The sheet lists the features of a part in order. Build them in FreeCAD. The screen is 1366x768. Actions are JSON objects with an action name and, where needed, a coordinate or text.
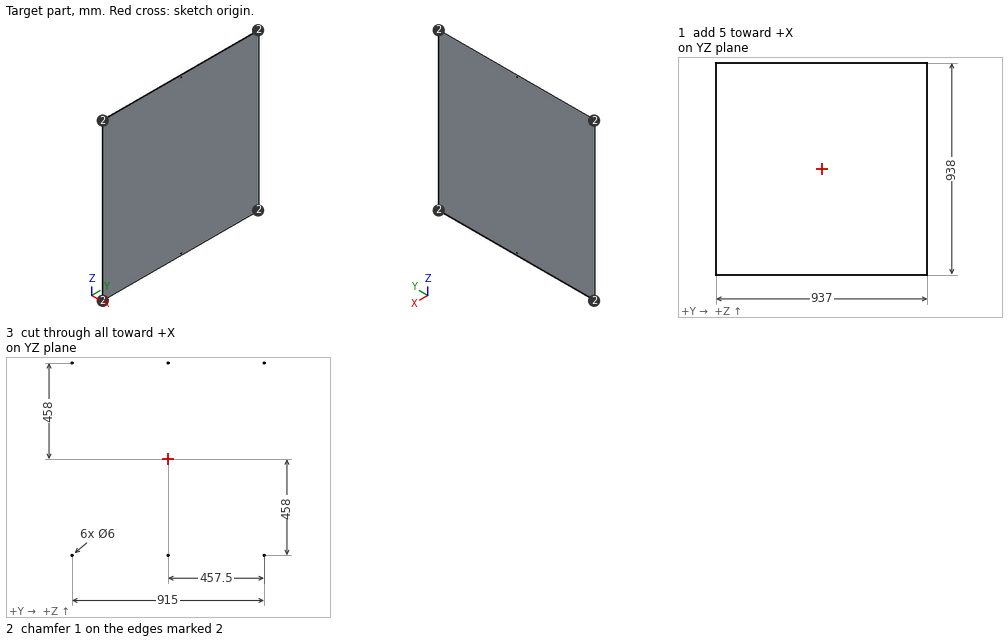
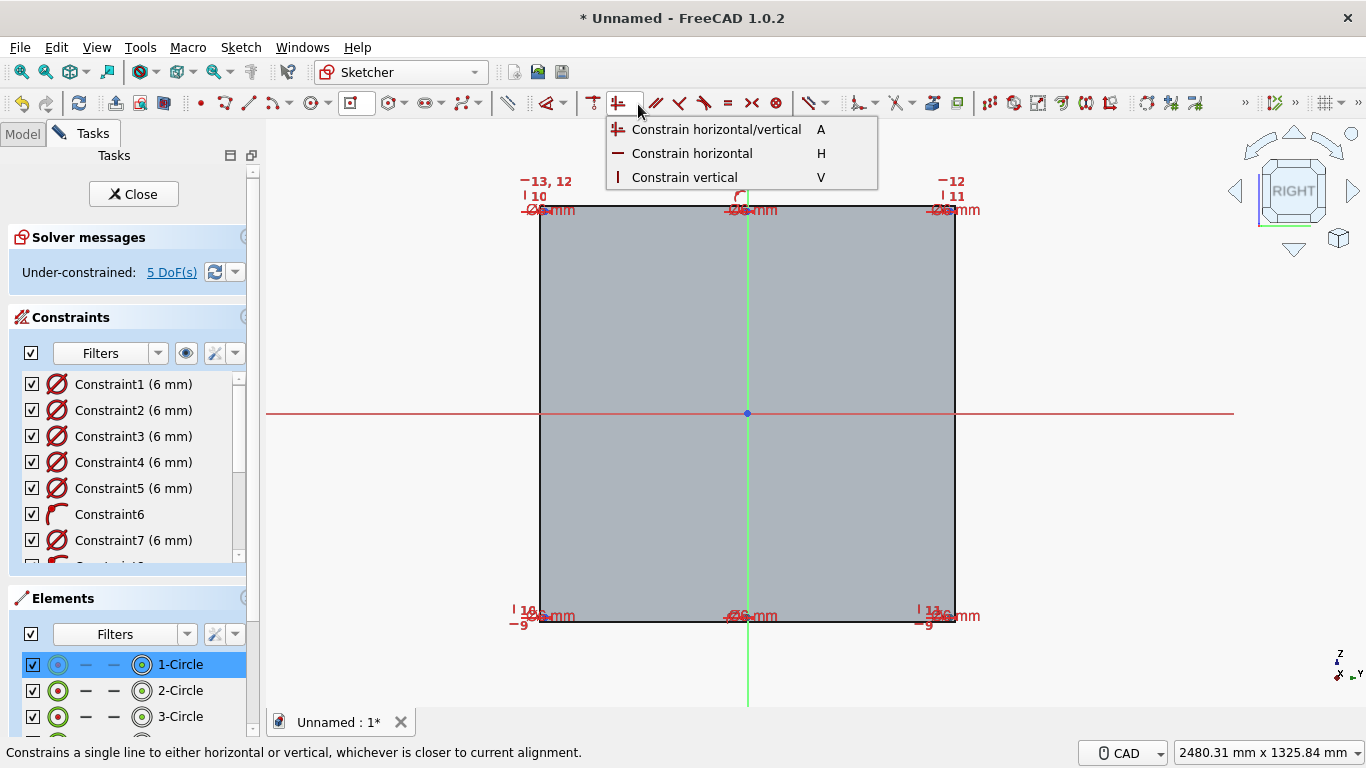
{"action": "left_click", "coordinate": [742, 153]}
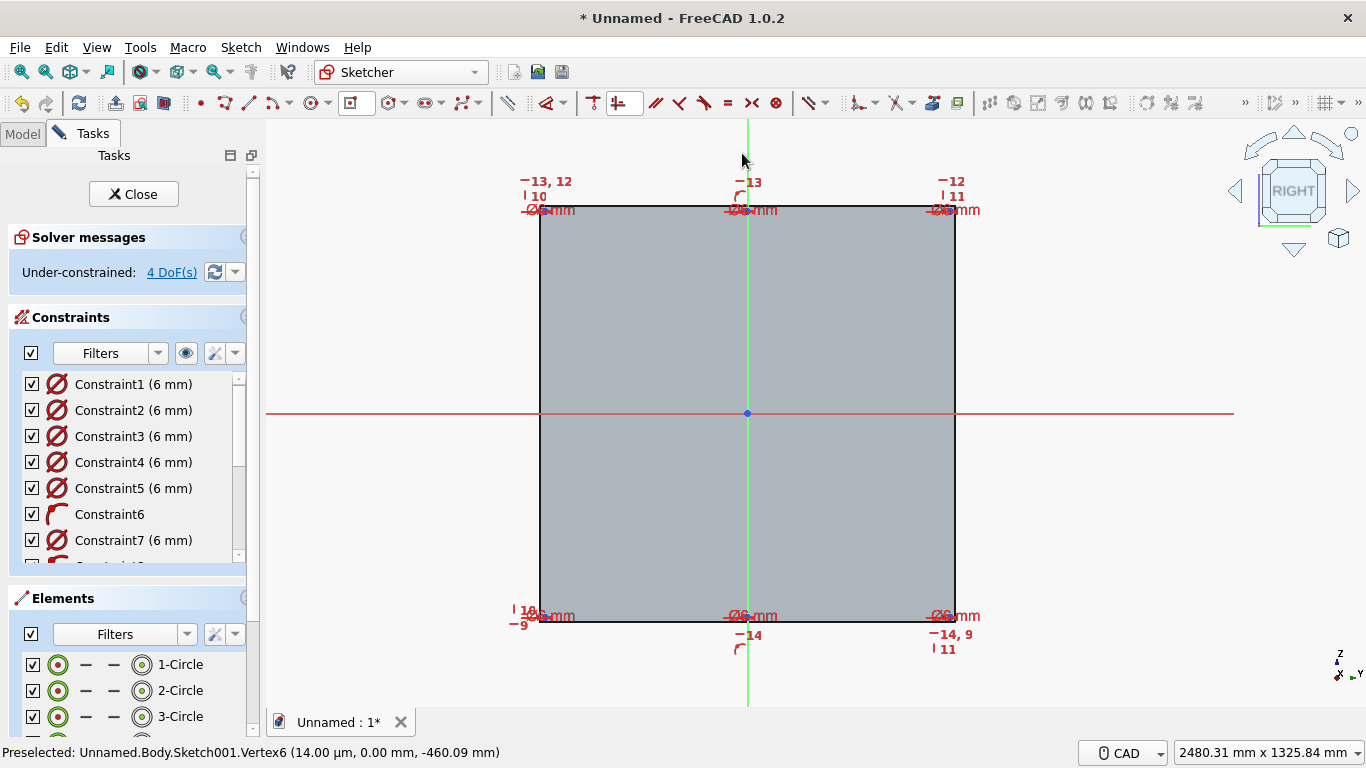
{"action": "left_click", "coordinate": [546, 104]}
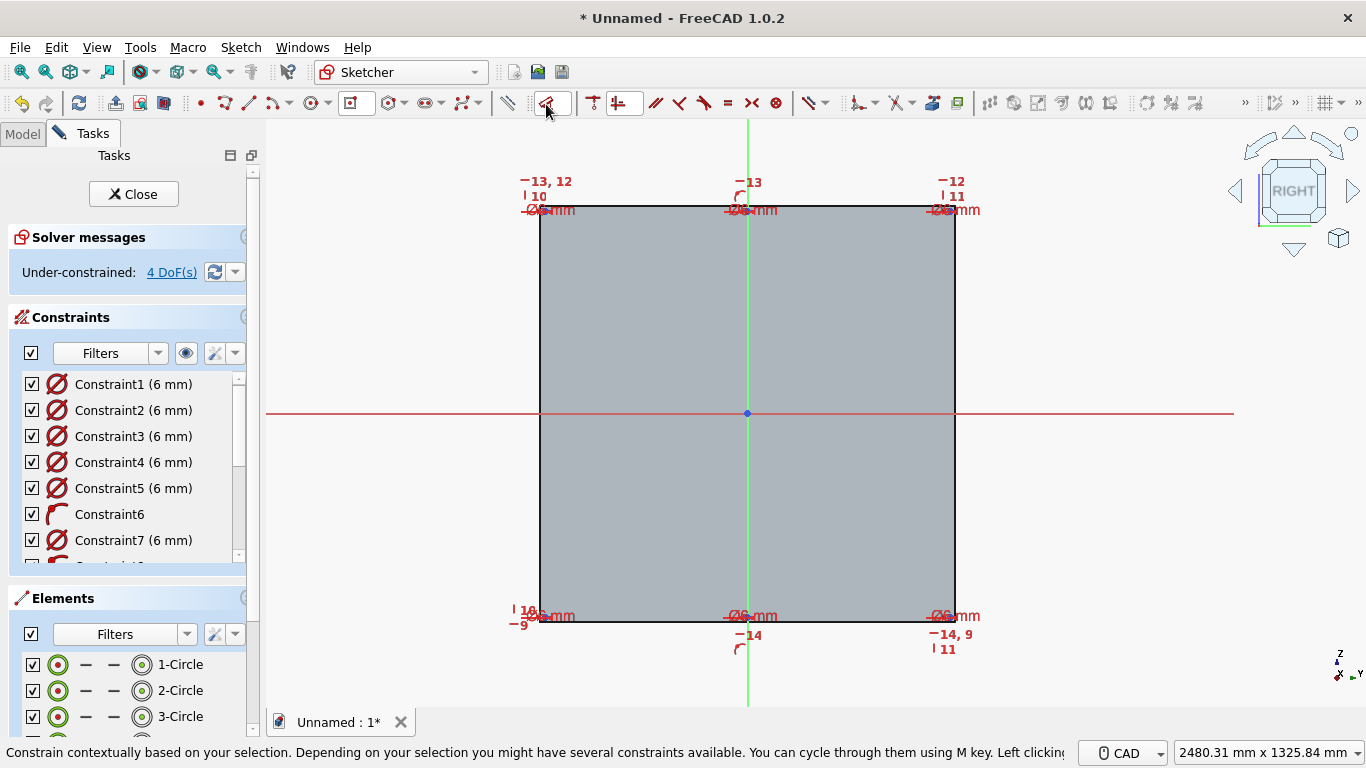
{"action": "left_click", "coordinate": [950, 618]}
{"action": "left_click", "coordinate": [984, 516]}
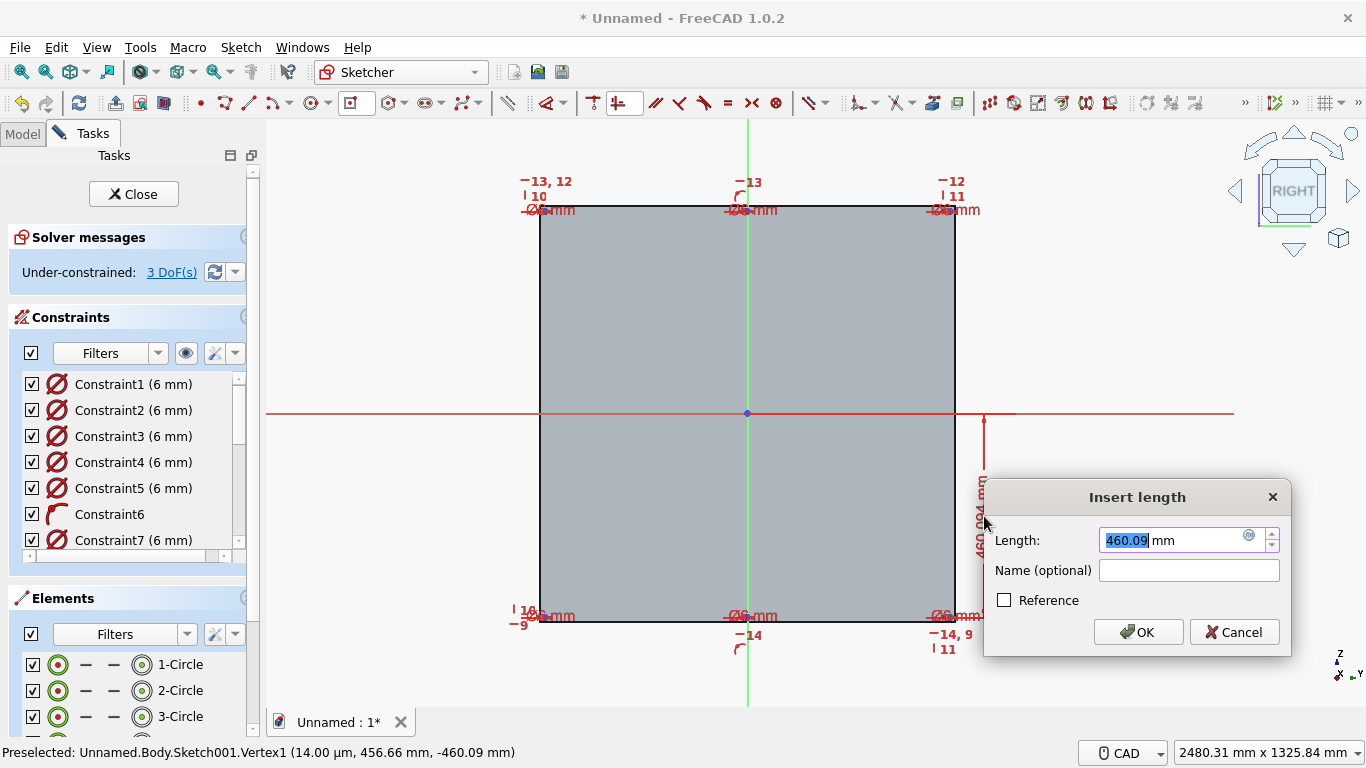
{"action": "type", "text": "458"}
{"action": "key", "text": "Return"}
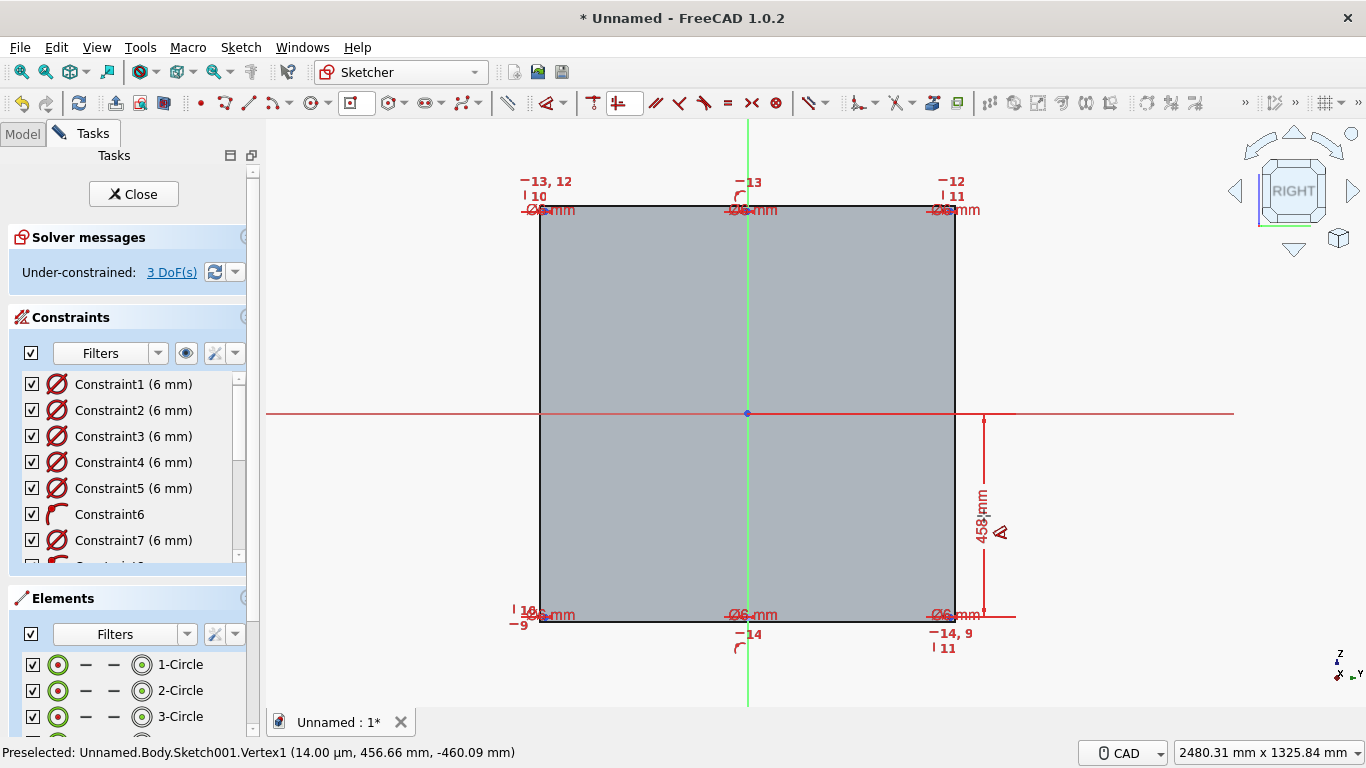
{"action": "left_click", "coordinate": [545, 212]}
{"action": "left_click", "coordinate": [511, 313]}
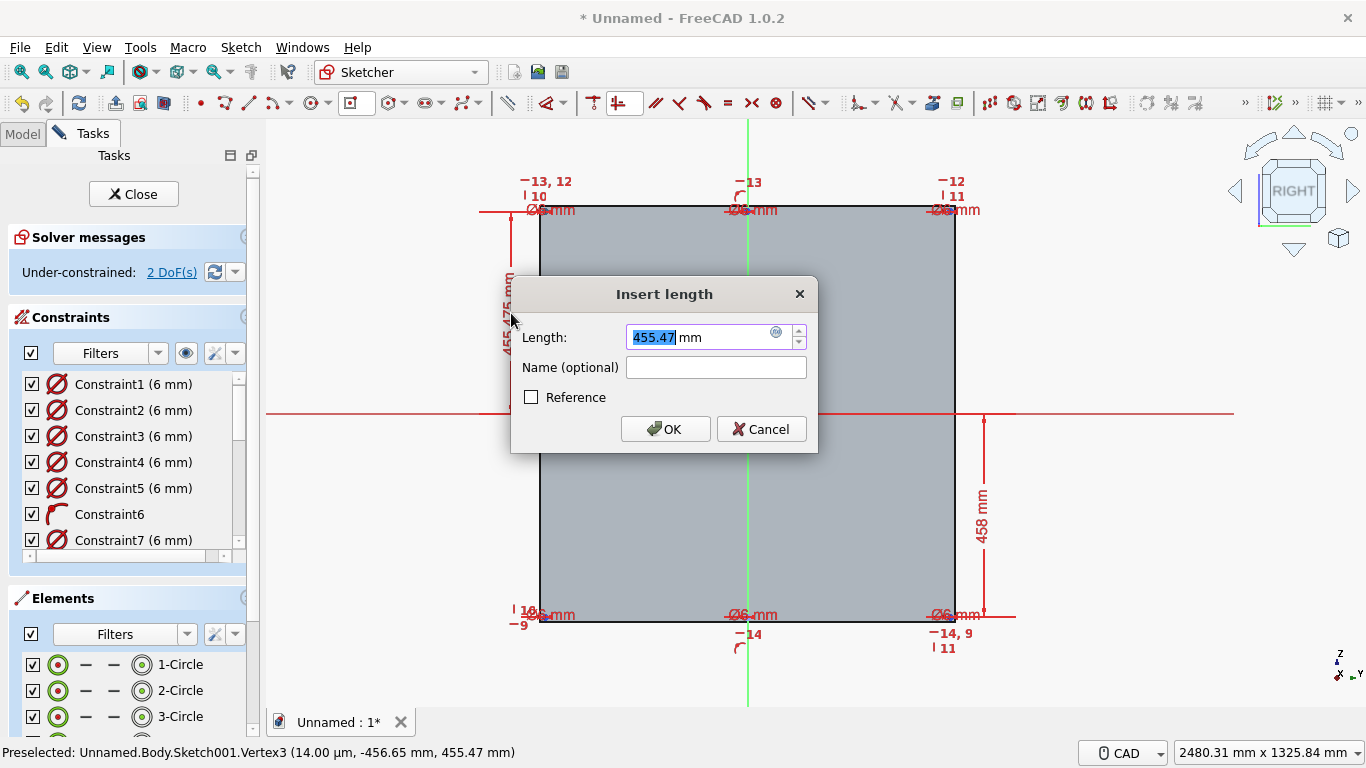
{"action": "type", "text": "458"}
{"action": "key", "text": "Return"}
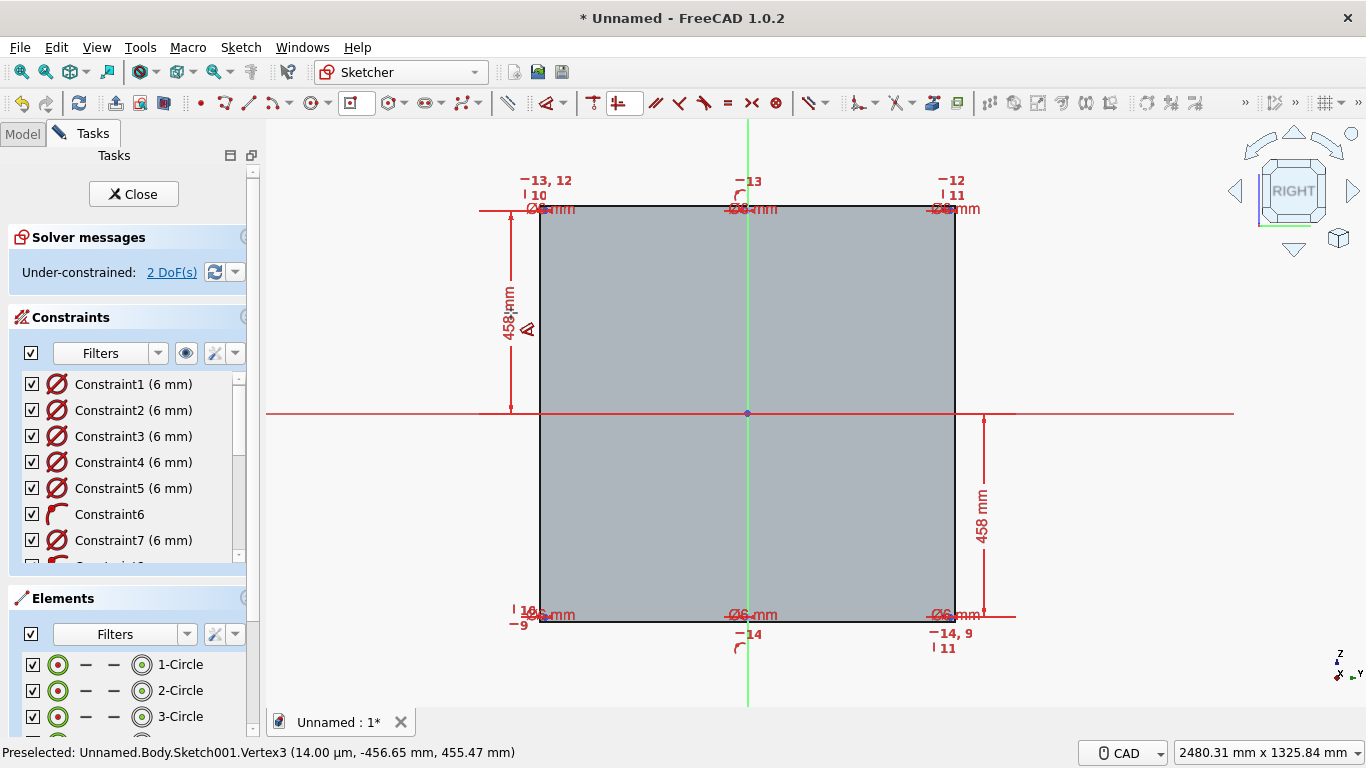
{"action": "left_click", "coordinate": [950, 617]}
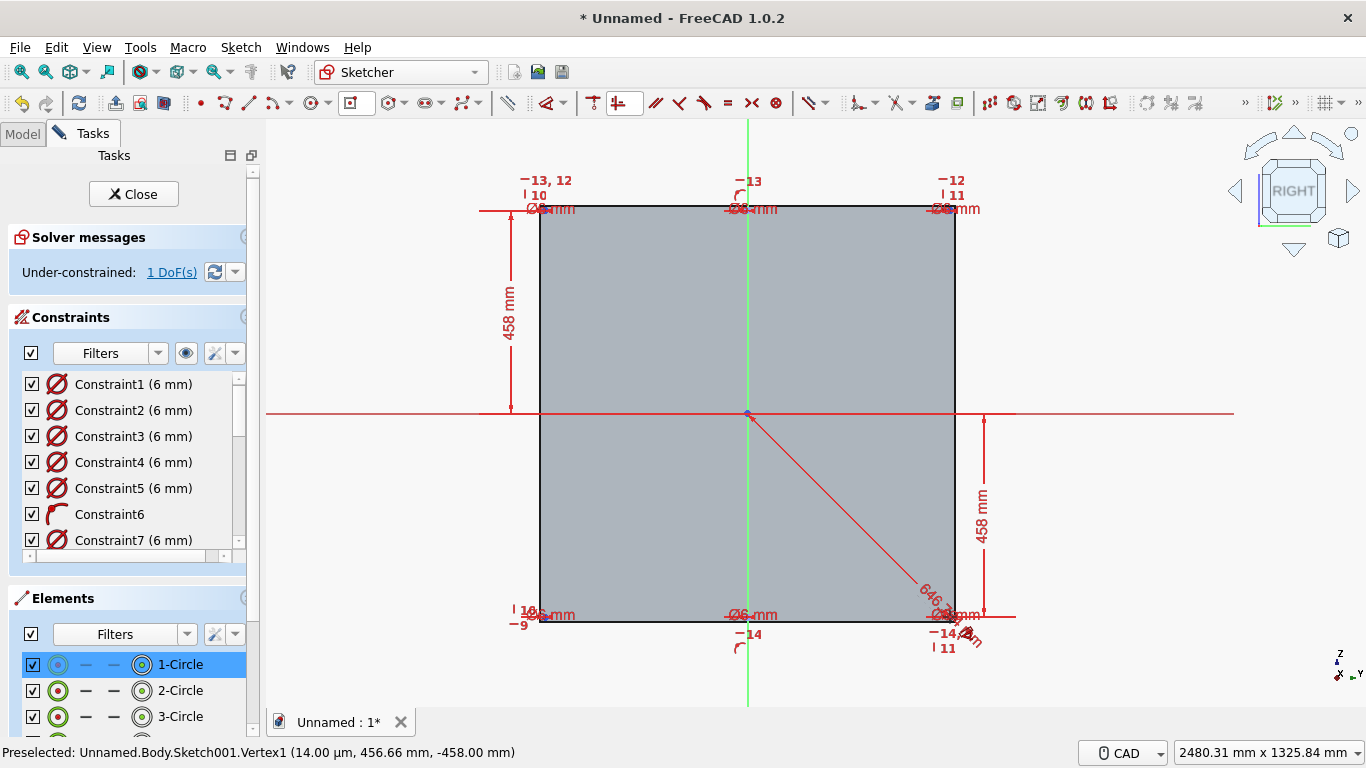
{"action": "left_click", "coordinate": [545, 617]}
{"action": "left_click", "coordinate": [654, 651]}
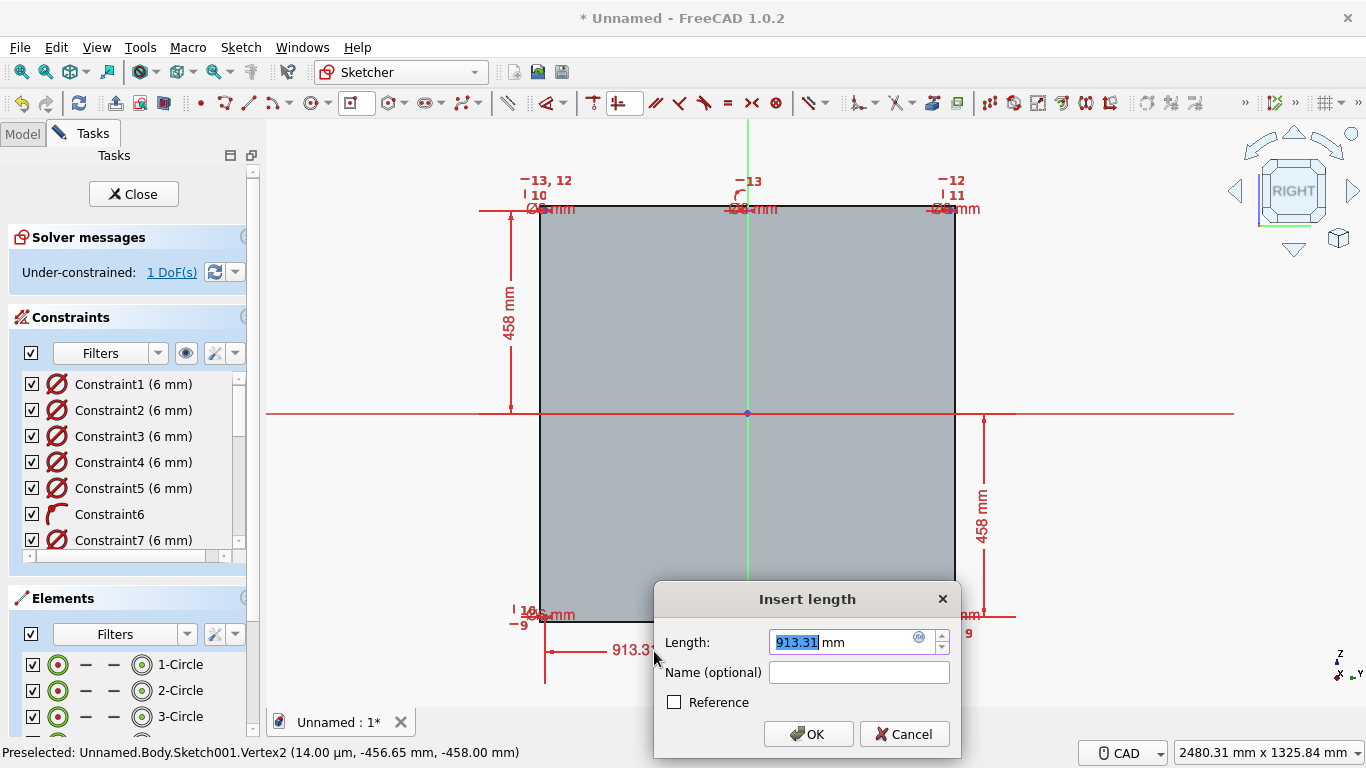
{"action": "type", "text": "915"}
{"action": "key", "text": "Return"}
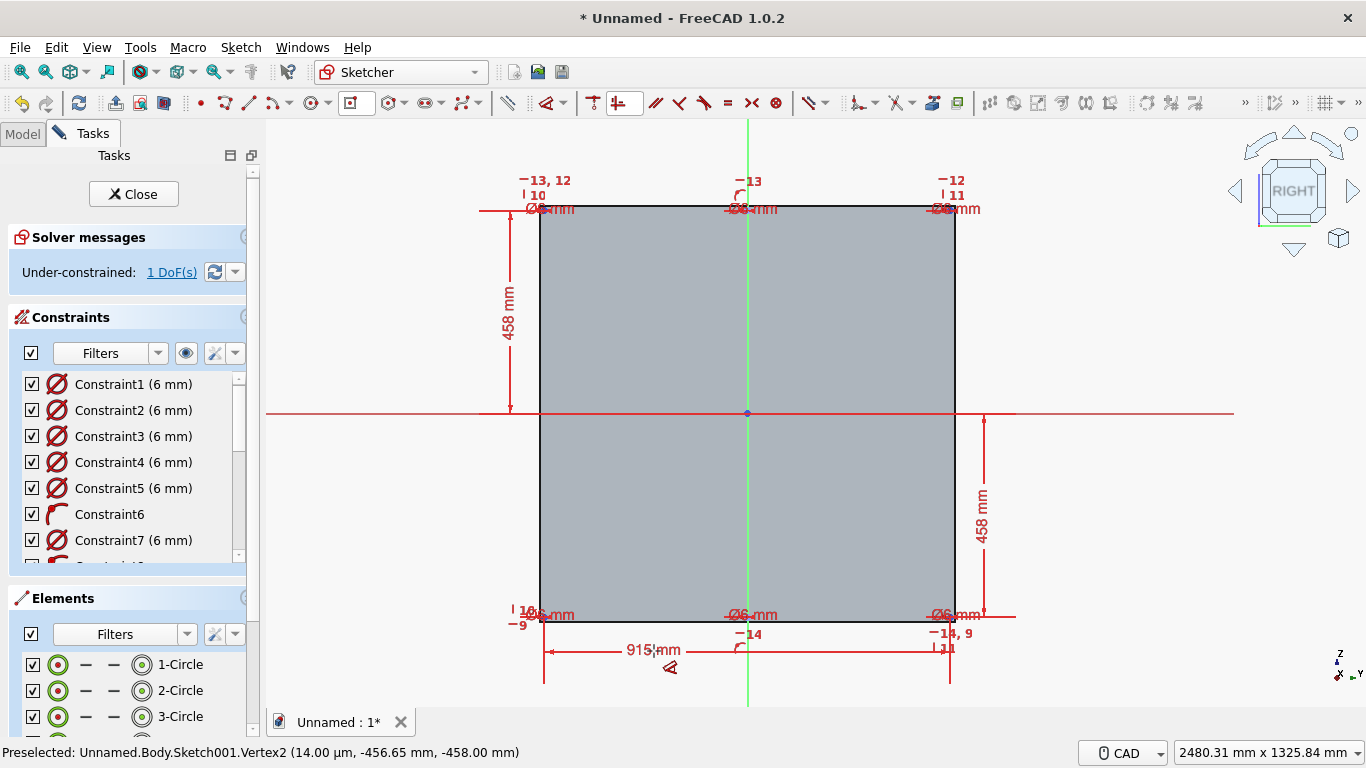
{"action": "left_click", "coordinate": [950, 617]}
{"action": "left_click", "coordinate": [849, 651]}